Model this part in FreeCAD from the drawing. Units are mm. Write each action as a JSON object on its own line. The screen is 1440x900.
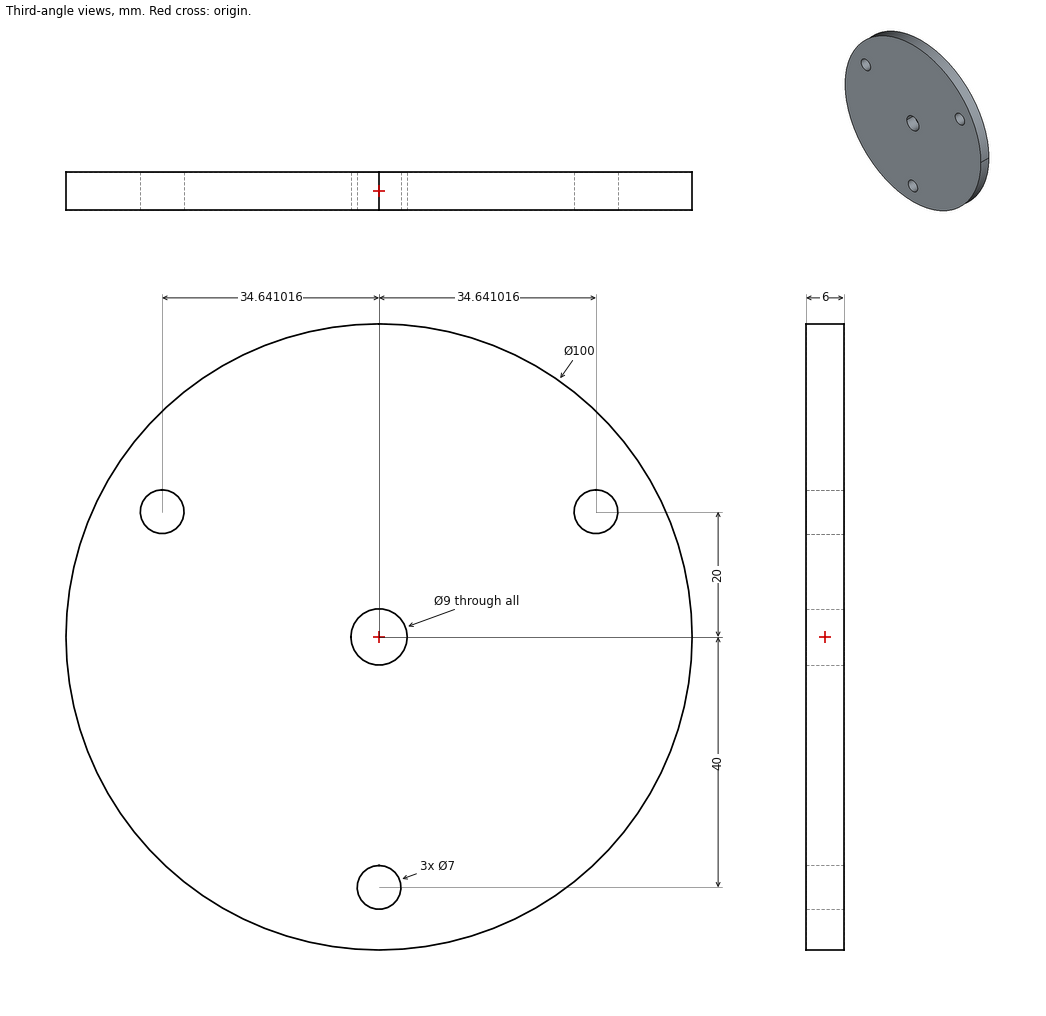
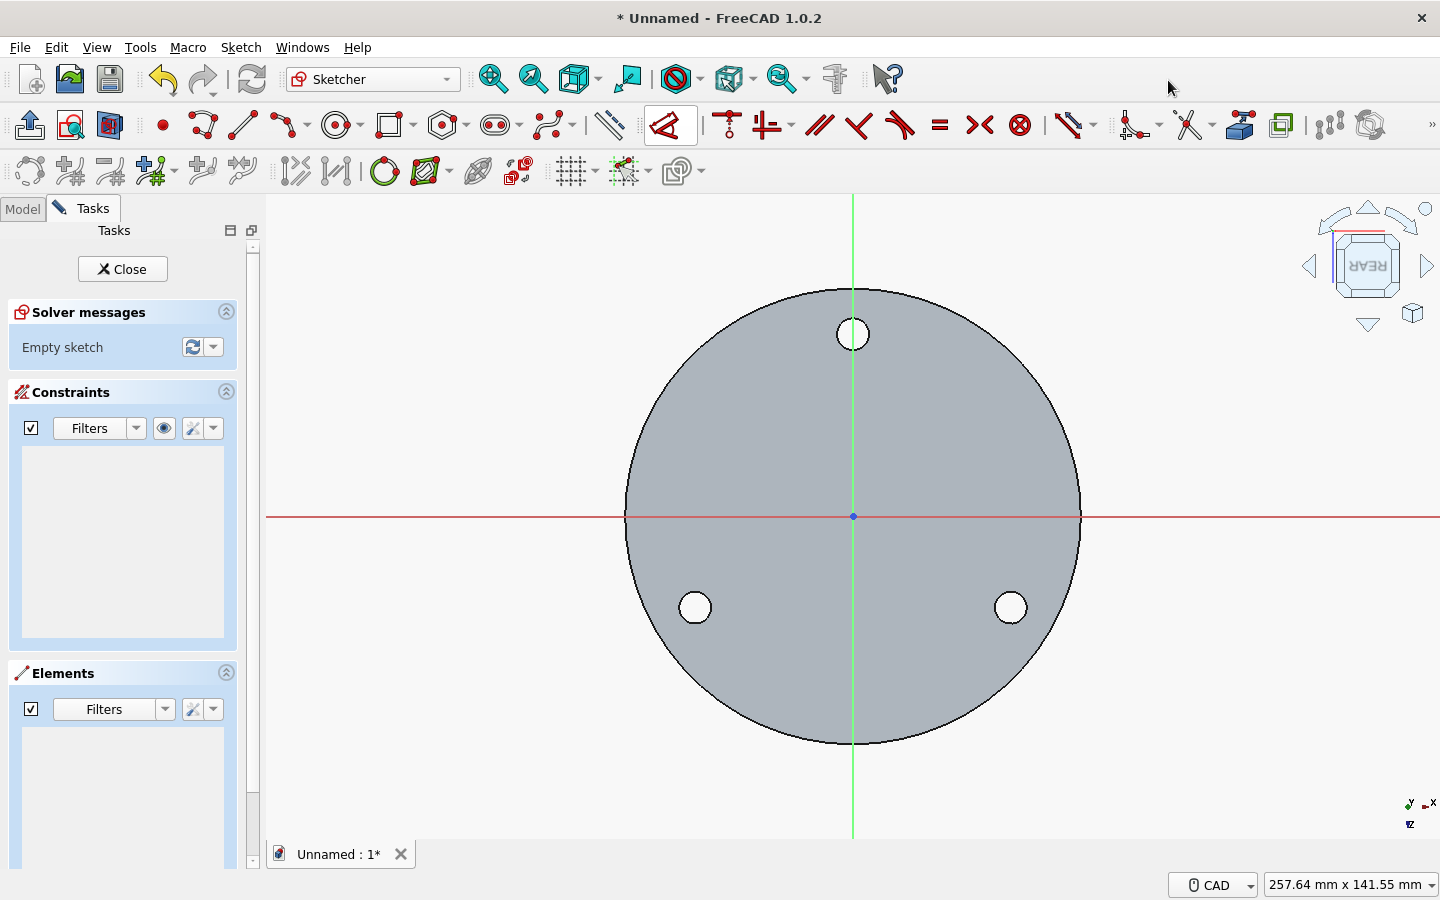
{"action": "scroll", "coordinate": [860, 516], "scroll_direction": "up", "scroll_amount": 12}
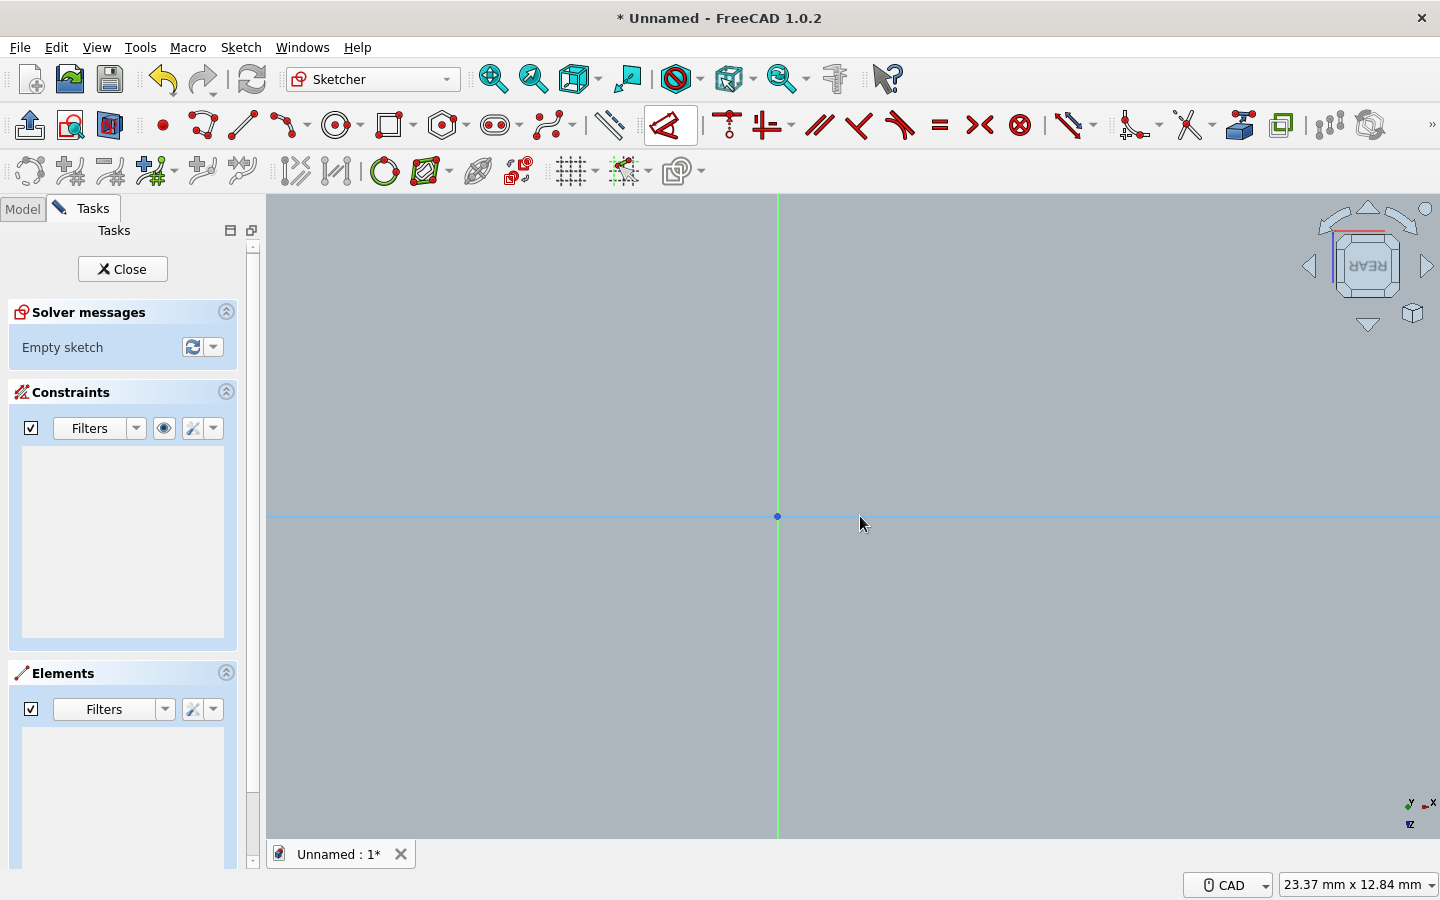
{"action": "left_click", "coordinate": [336, 126]}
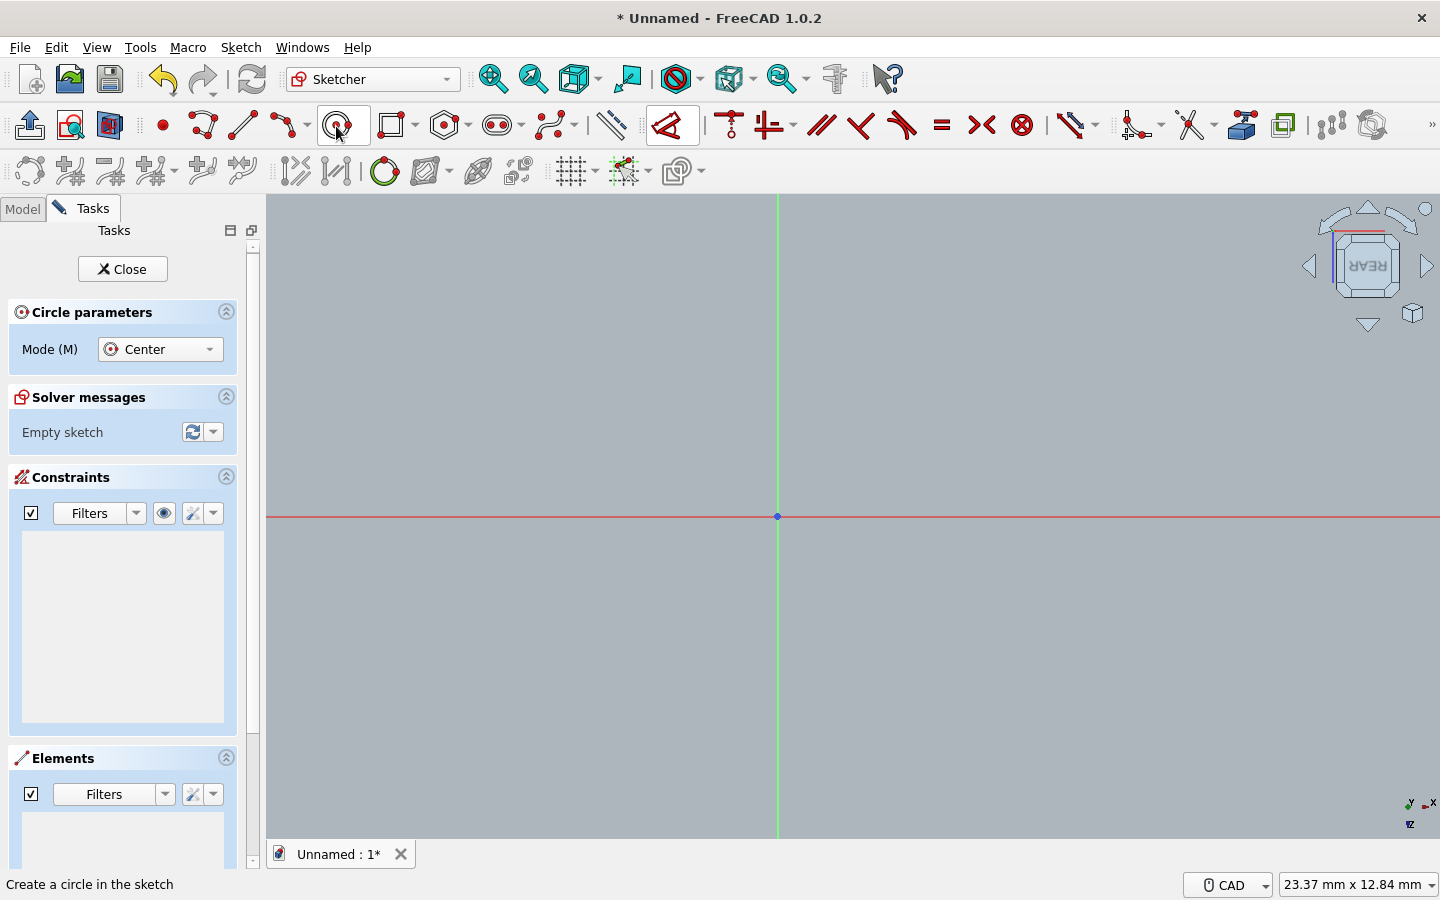
{"action": "left_click", "coordinate": [778, 516]}
{"action": "mouse_move", "coordinate": [938, 357]}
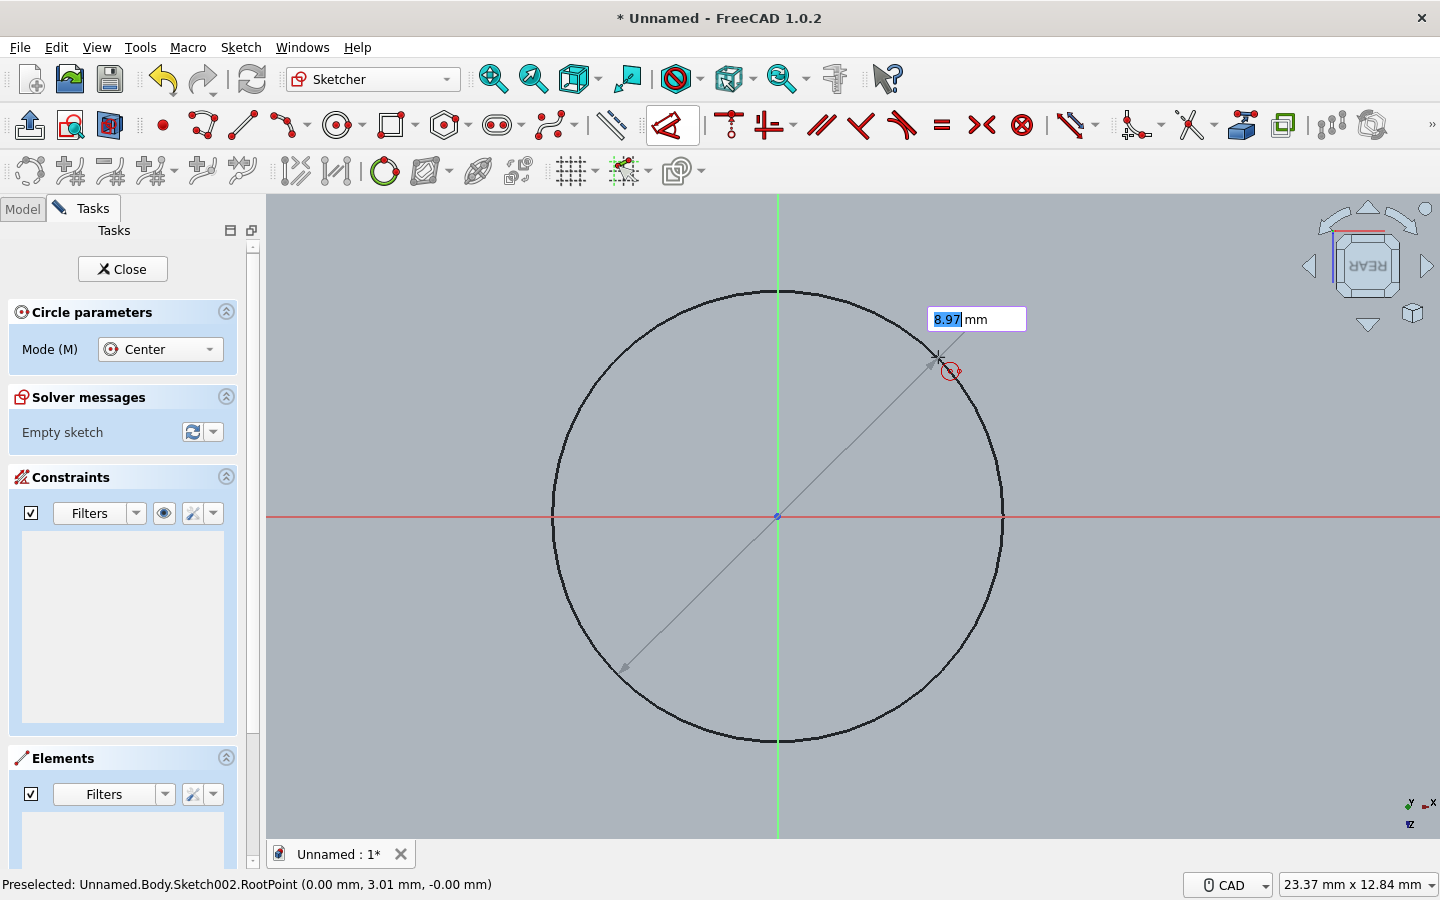
{"action": "type", "text": "9"}
{"action": "key", "text": "Return"}
{"action": "key", "text": "Escape"}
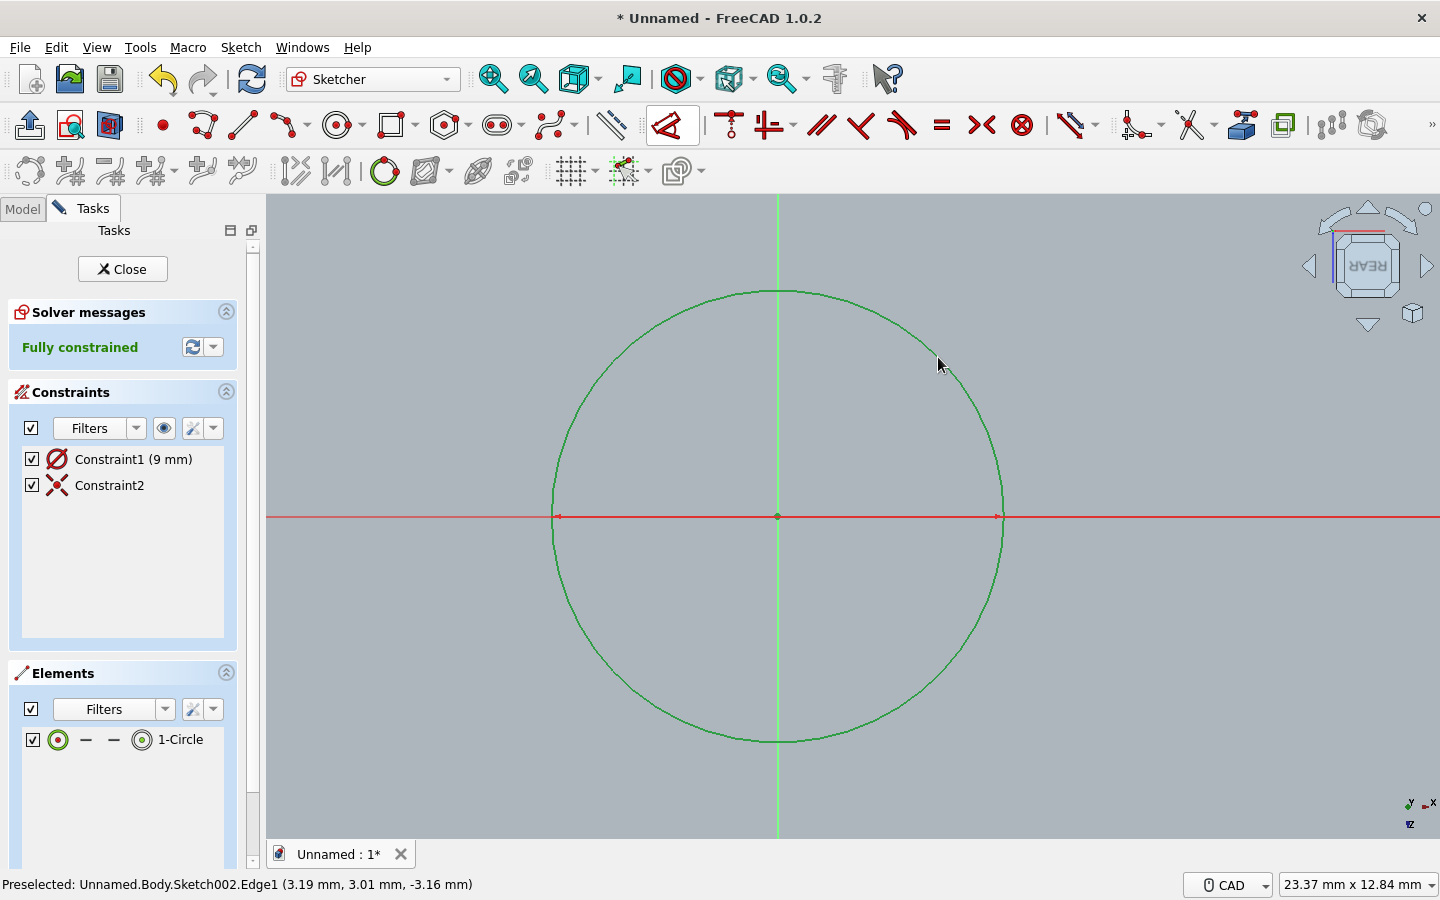
{"action": "left_click", "coordinate": [123, 269]}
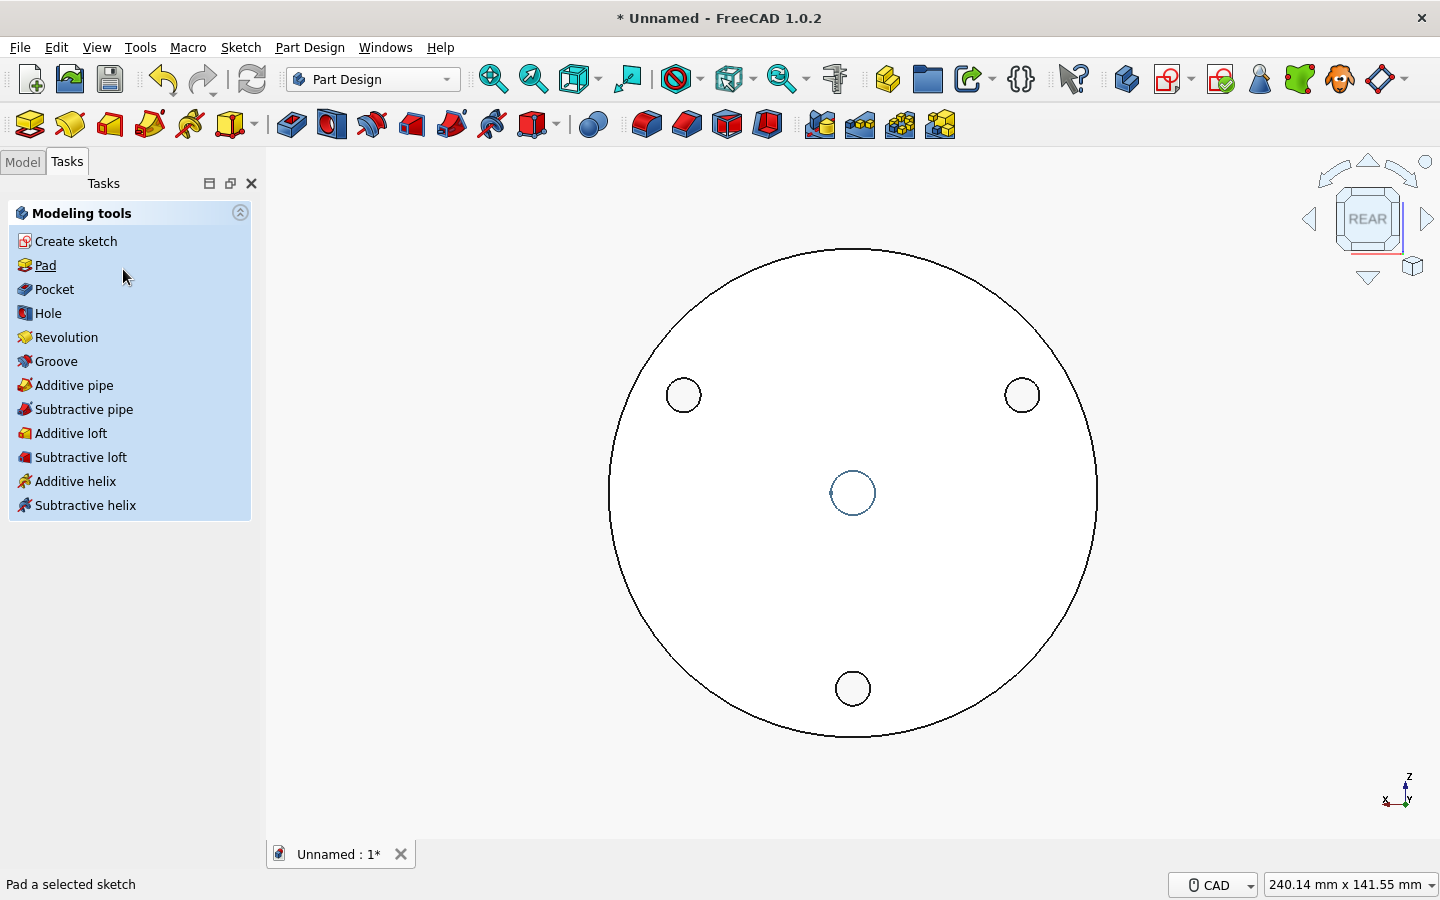
{"action": "left_click", "coordinate": [332, 124]}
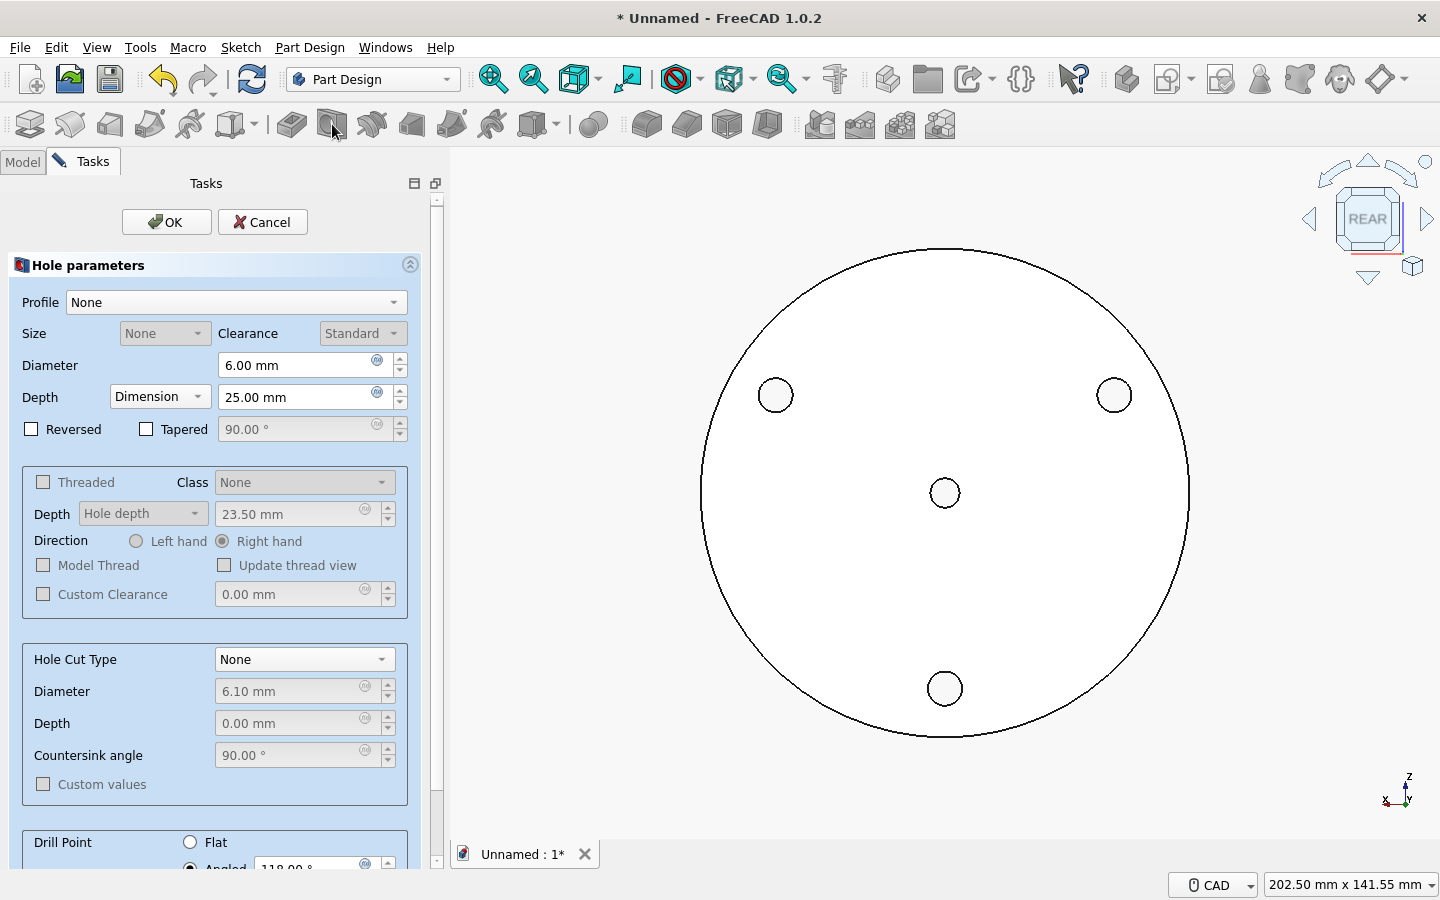
{"action": "triple_click", "coordinate": [305, 365]}